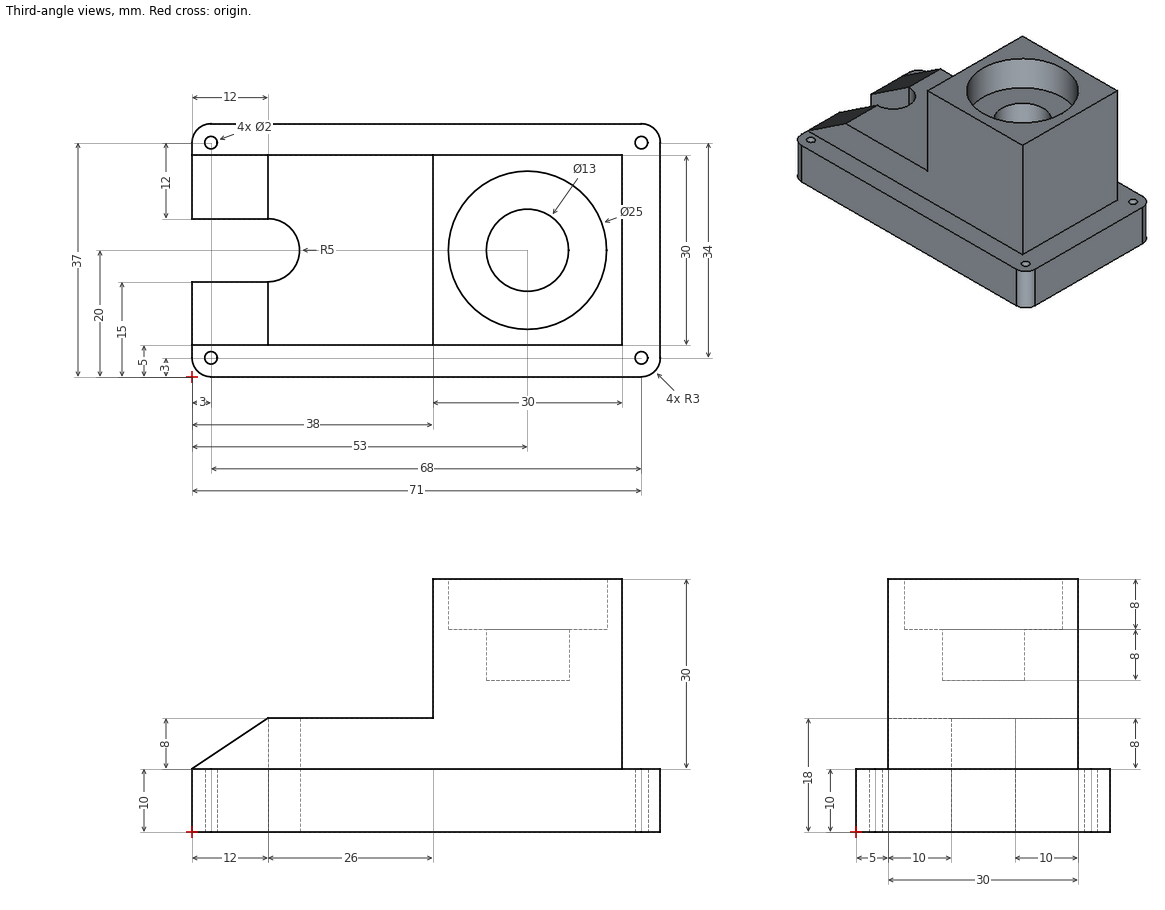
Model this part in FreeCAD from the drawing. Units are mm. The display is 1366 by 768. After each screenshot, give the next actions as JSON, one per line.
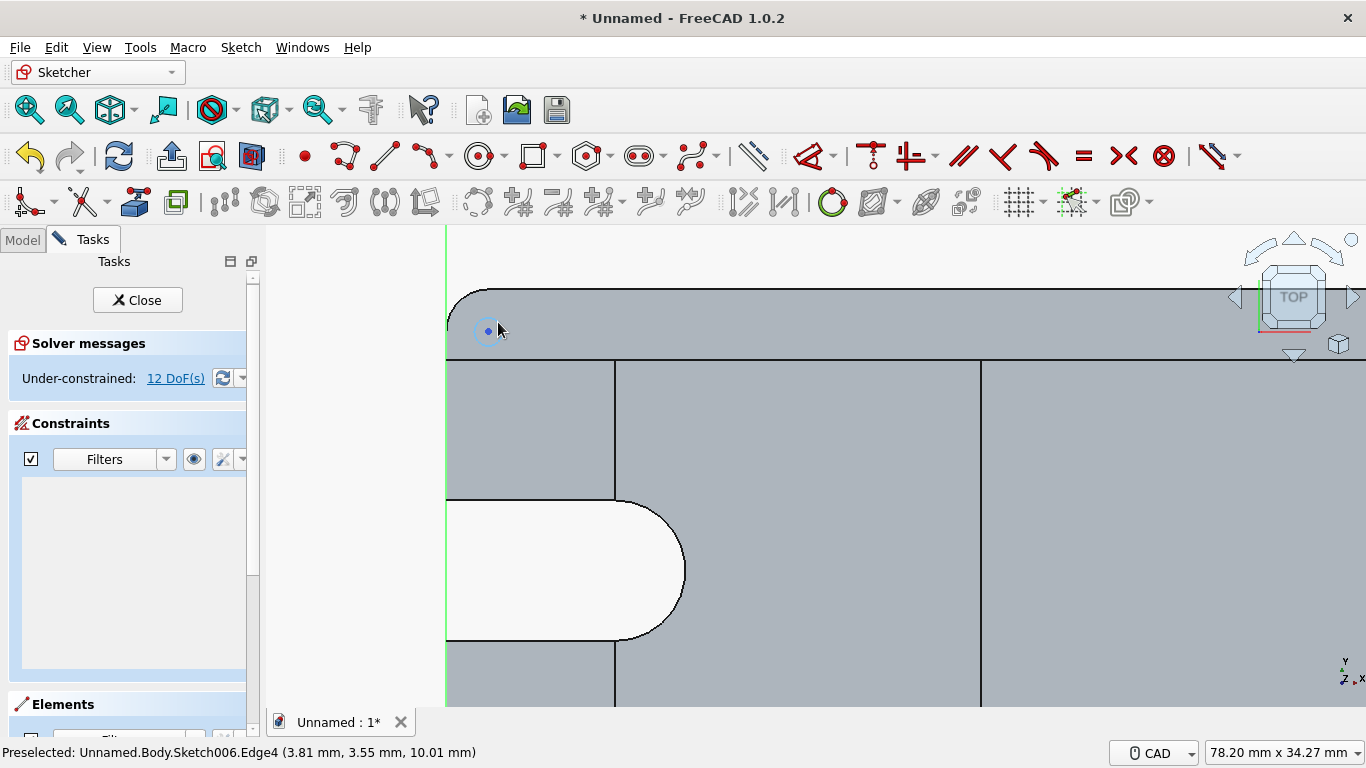
{"action": "left_click", "coordinate": [498, 322]}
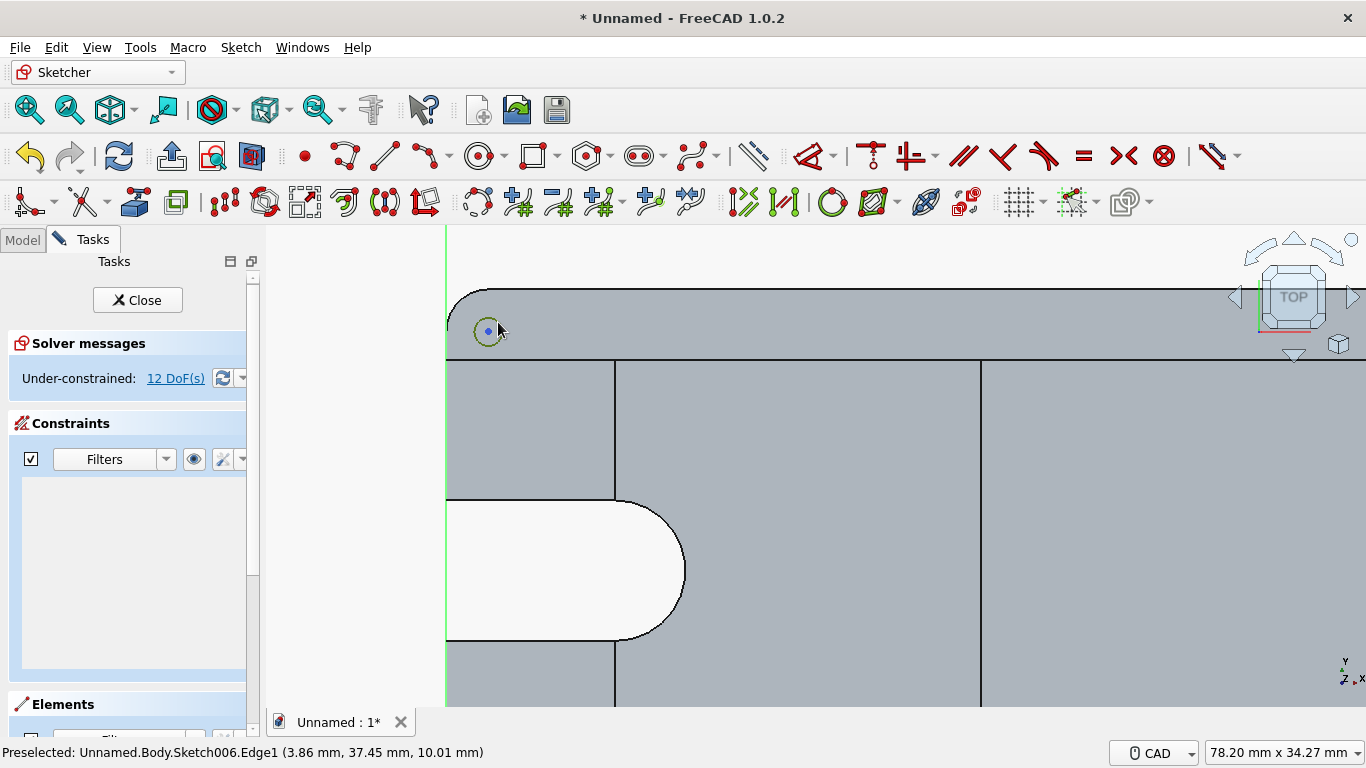
{"action": "scroll", "coordinate": [498, 322], "scroll_direction": "down", "scroll_amount": 3}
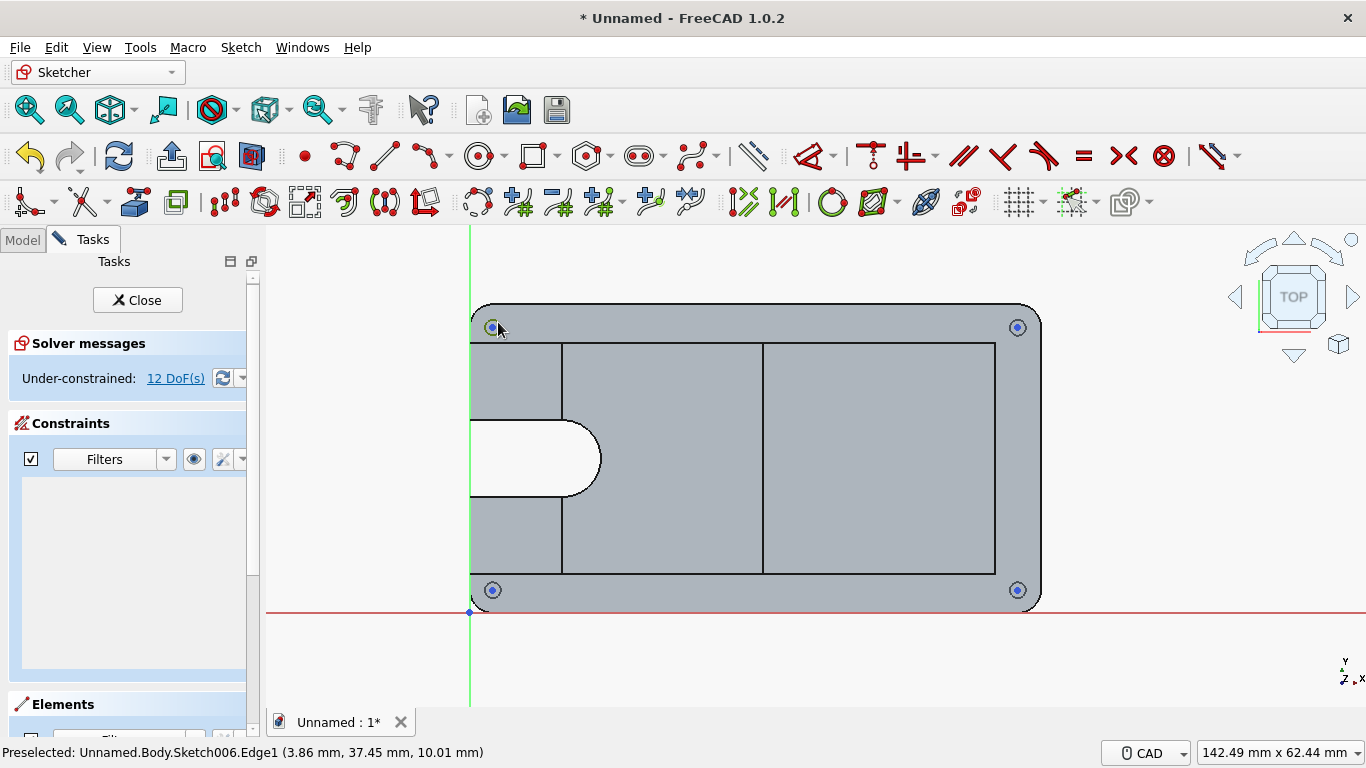
{"action": "scroll", "coordinate": [1023, 322], "scroll_direction": "up", "scroll_amount": 3}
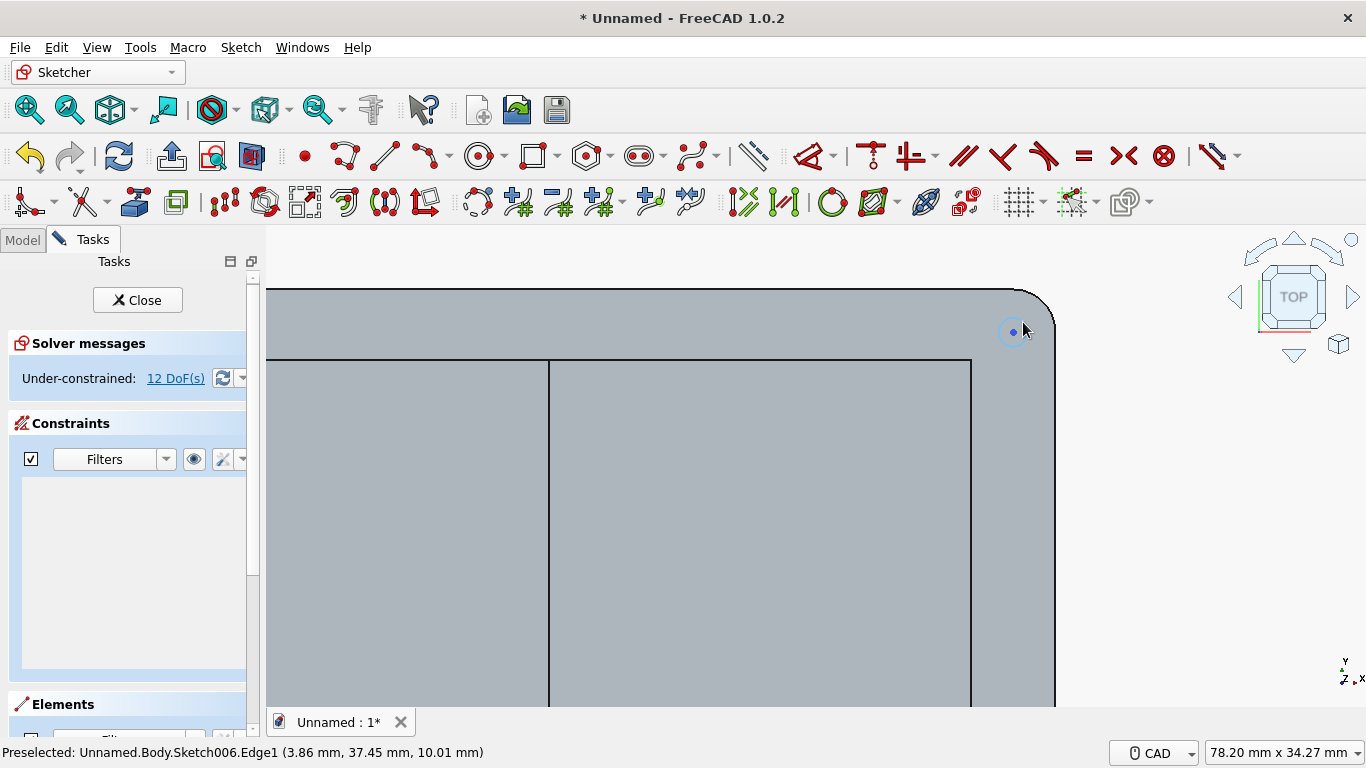
{"action": "left_click", "coordinate": [1023, 322]}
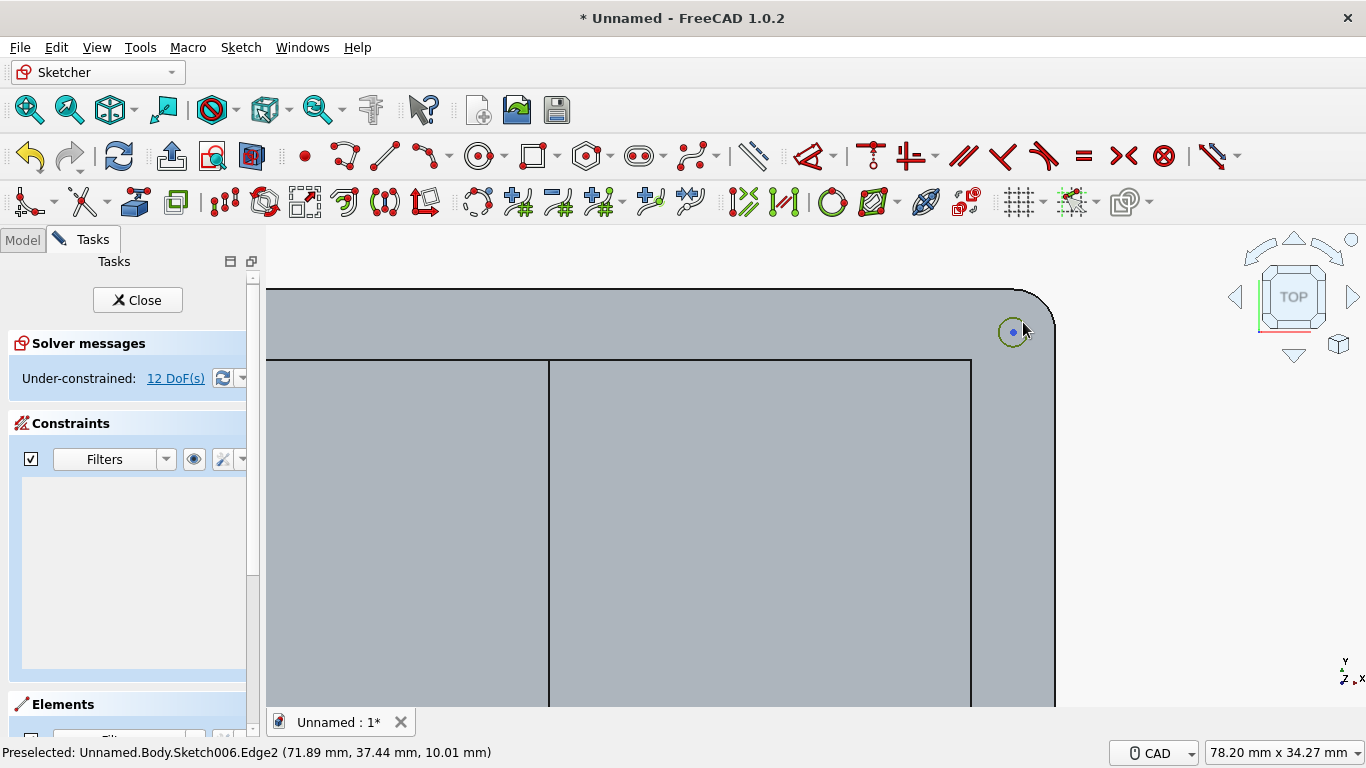
{"action": "scroll", "coordinate": [1023, 322], "scroll_direction": "down", "scroll_amount": 3}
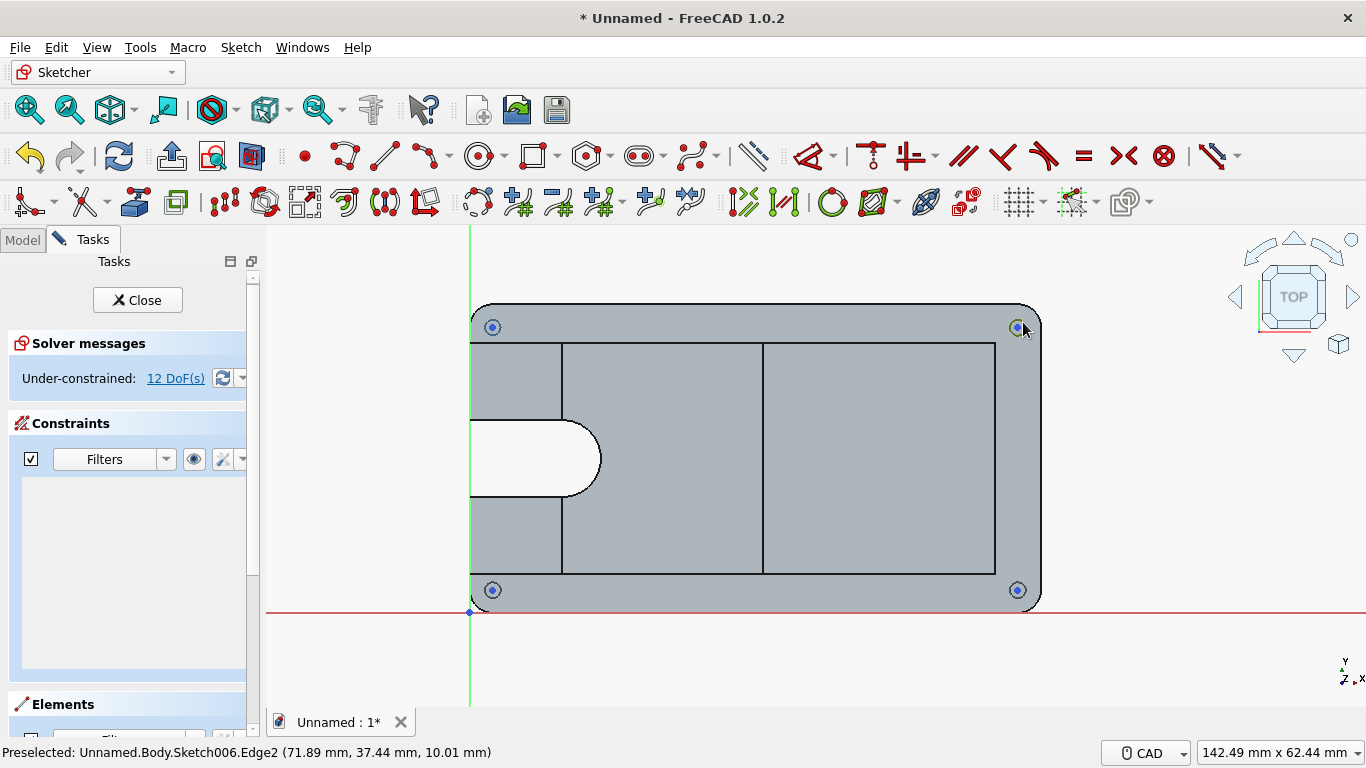
{"action": "scroll", "coordinate": [1023, 585], "scroll_direction": "up", "scroll_amount": 3}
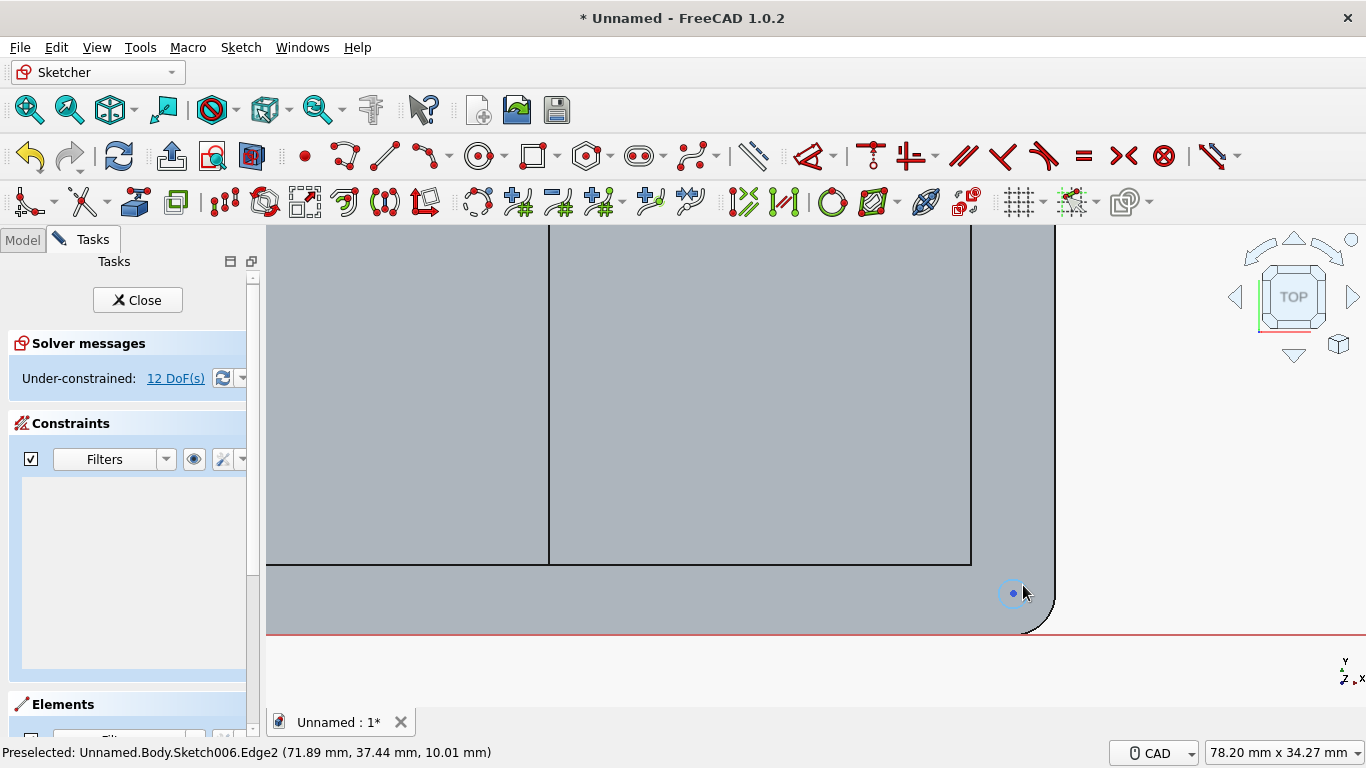
{"action": "left_click", "coordinate": [1023, 584]}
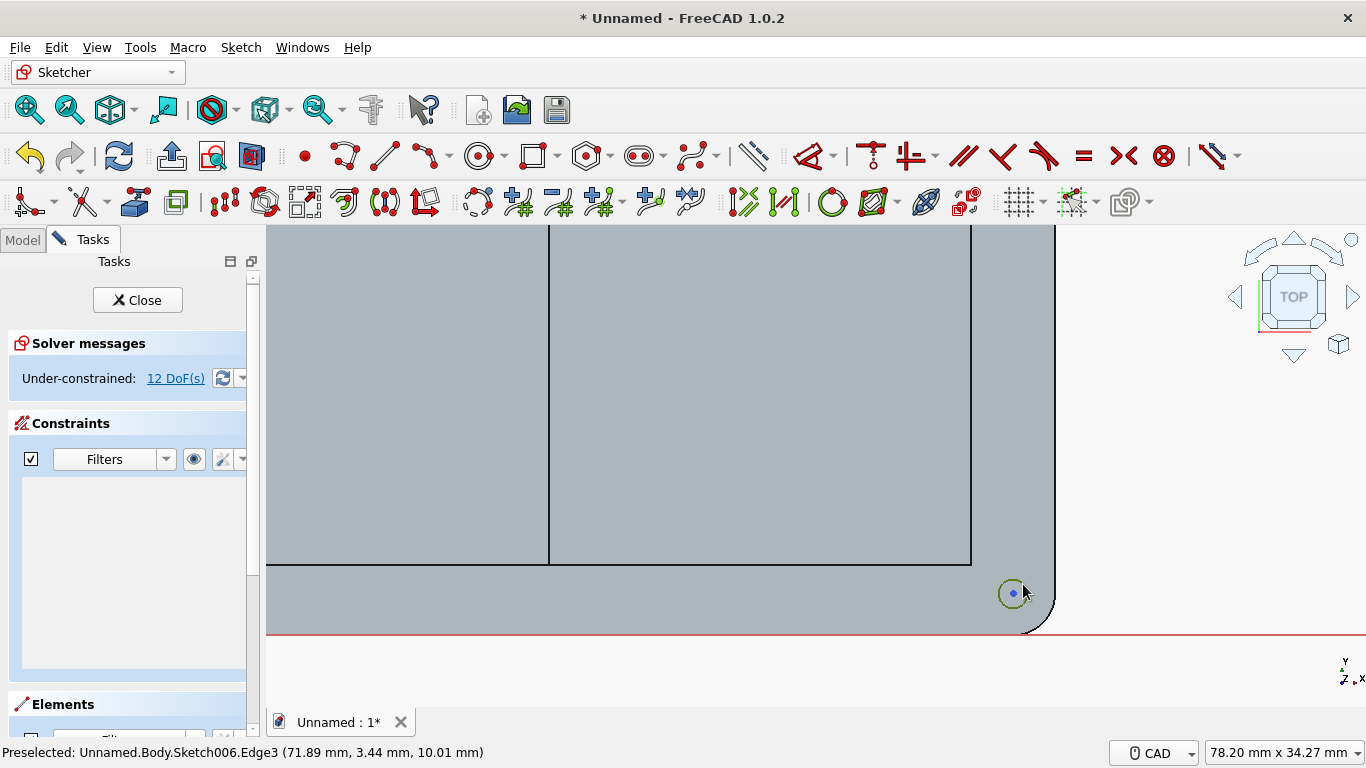
{"action": "scroll", "coordinate": [1023, 585], "scroll_direction": "down", "scroll_amount": 3}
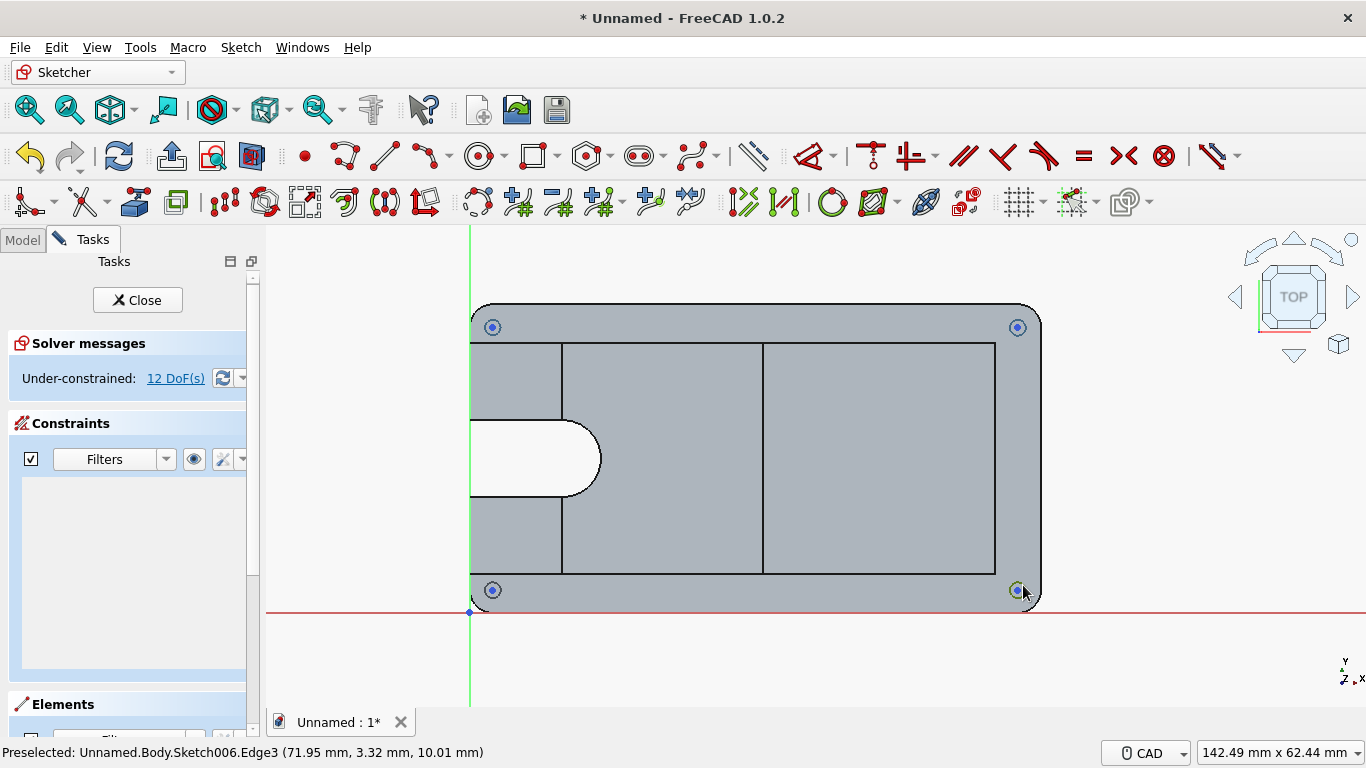
{"action": "scroll", "coordinate": [498, 585], "scroll_direction": "up", "scroll_amount": 3}